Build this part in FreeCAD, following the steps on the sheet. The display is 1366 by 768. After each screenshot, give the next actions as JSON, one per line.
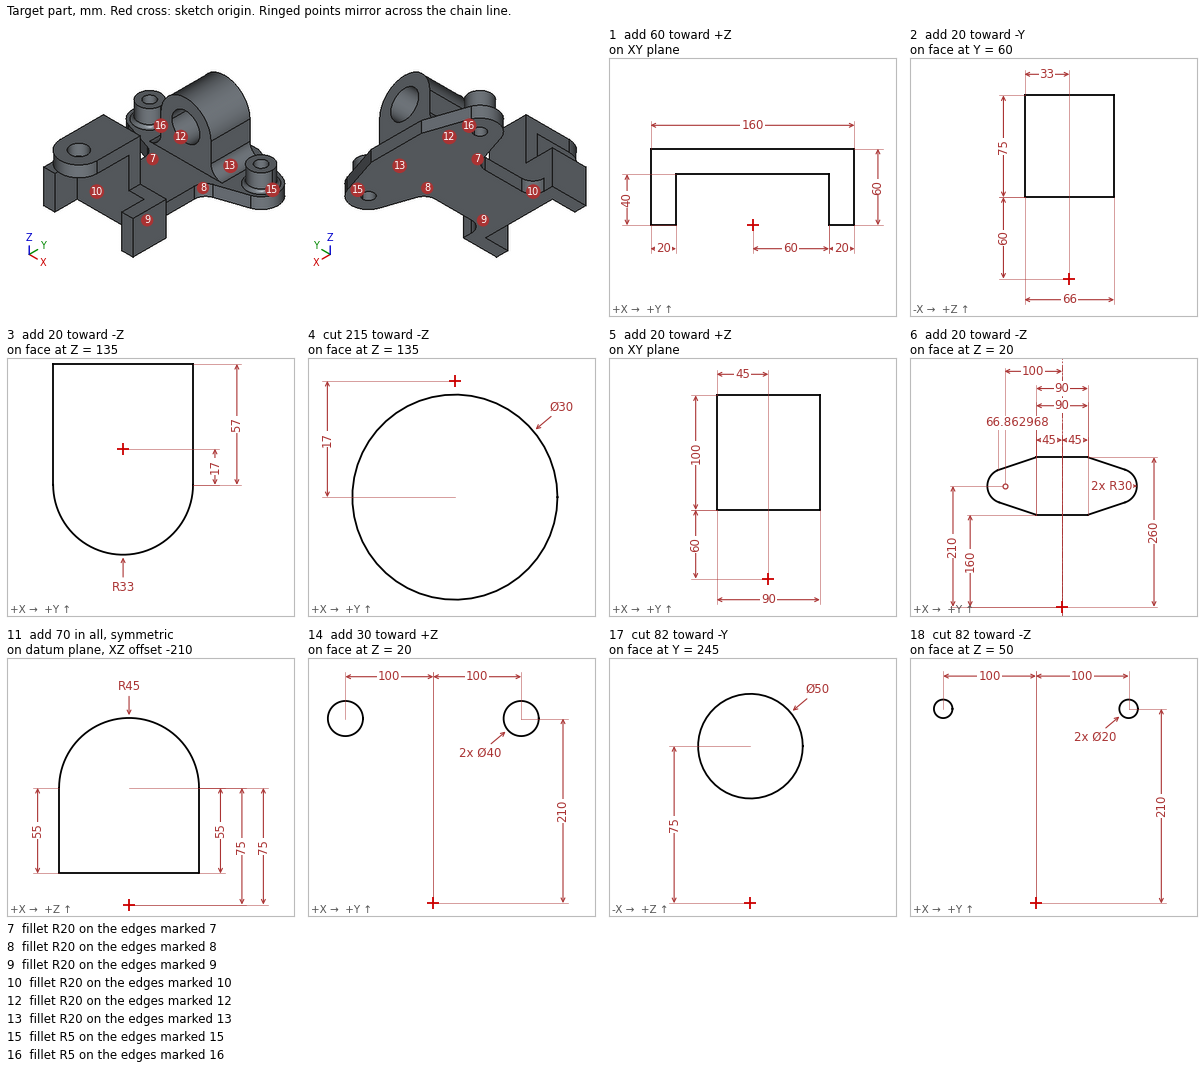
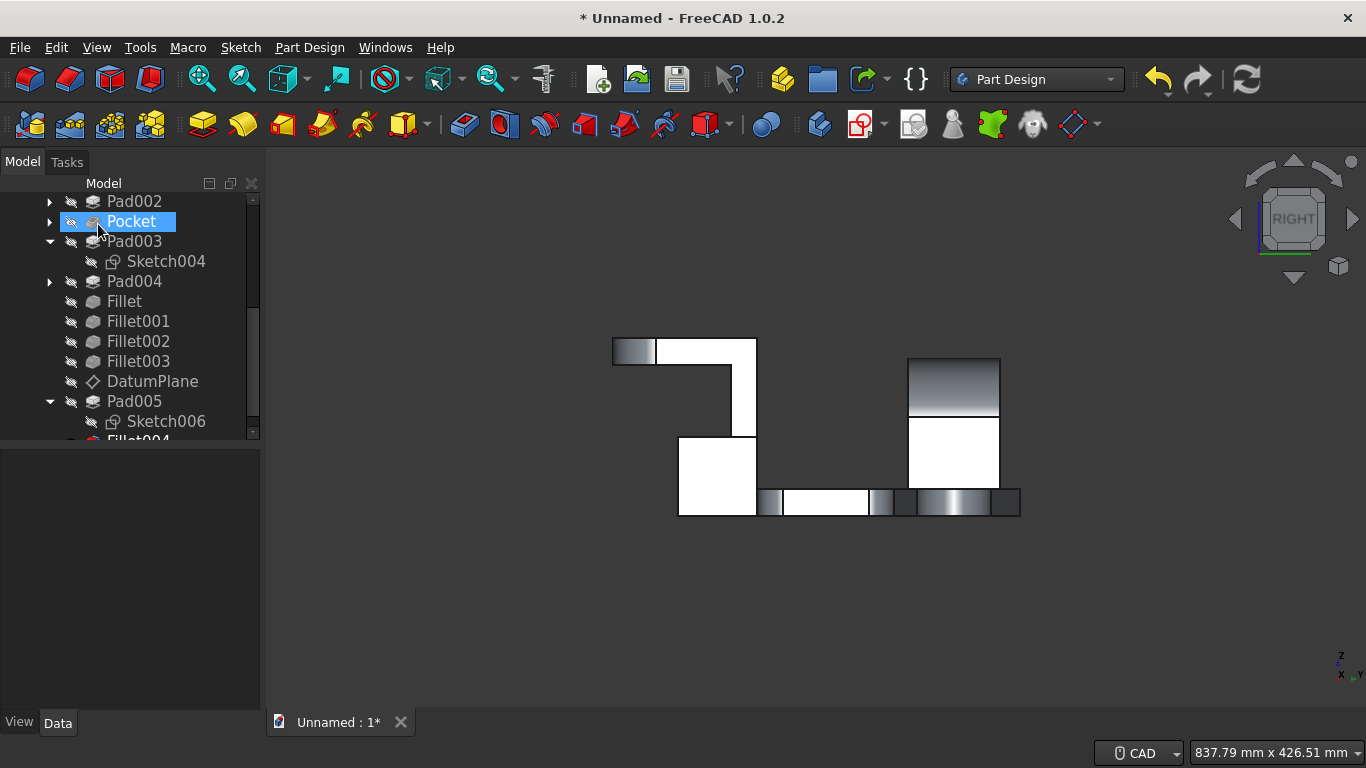
{"action": "key", "text": "v f"}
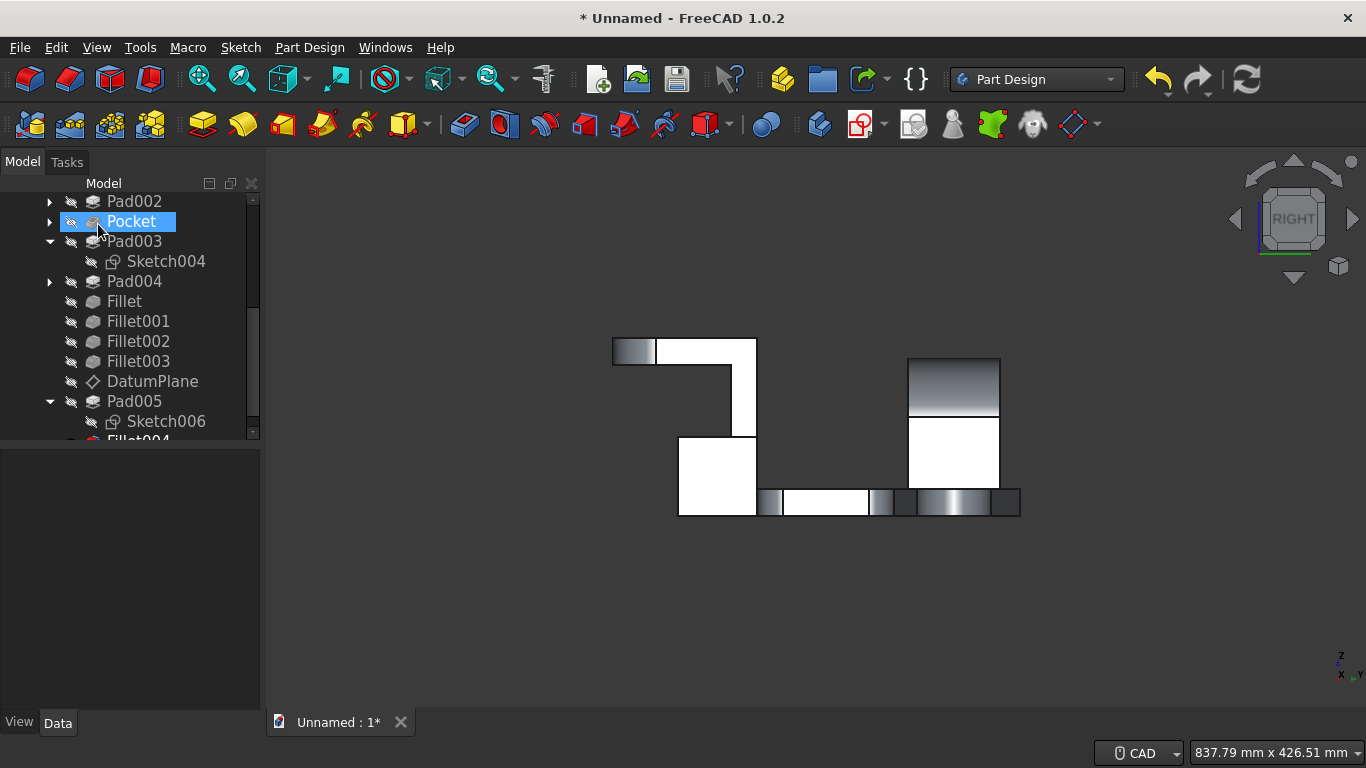
{"action": "key", "text": "5"}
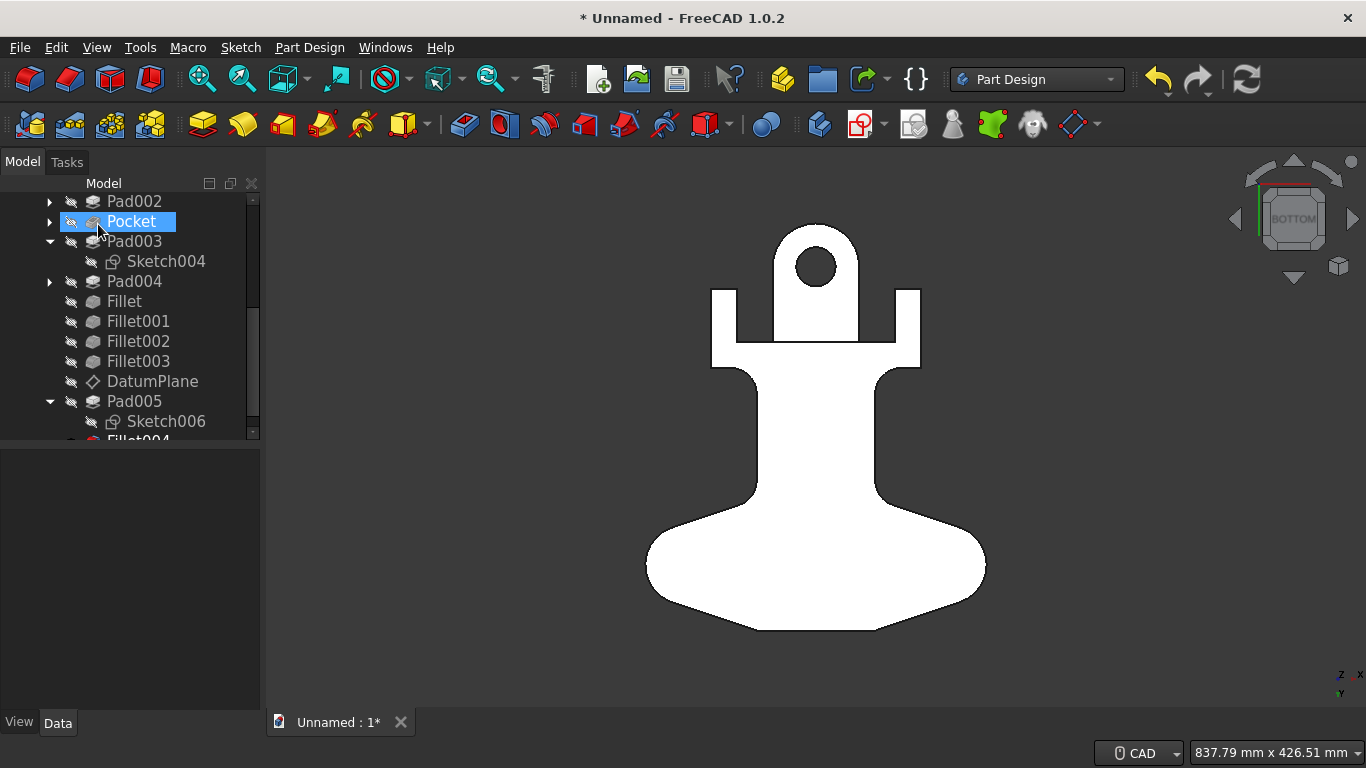
{"action": "key", "text": "4"}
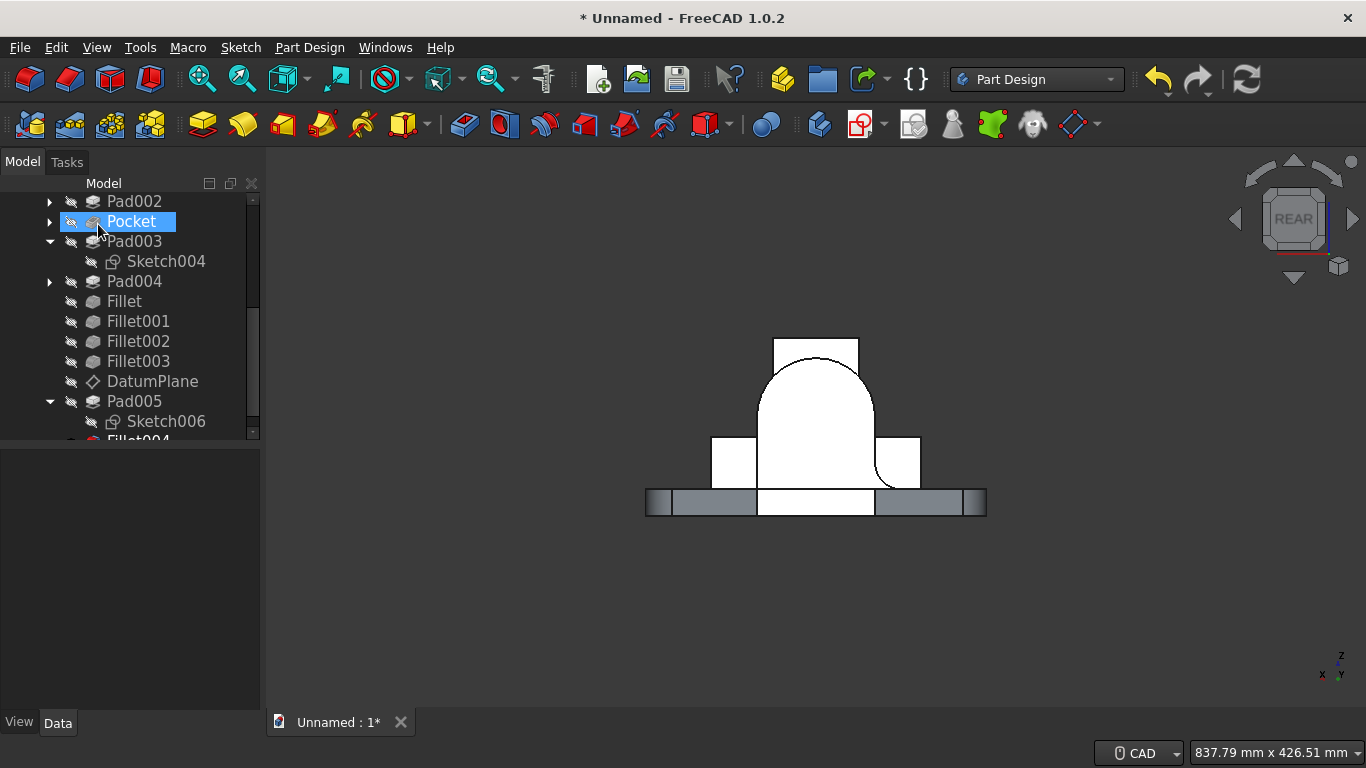
{"action": "key", "text": "v f"}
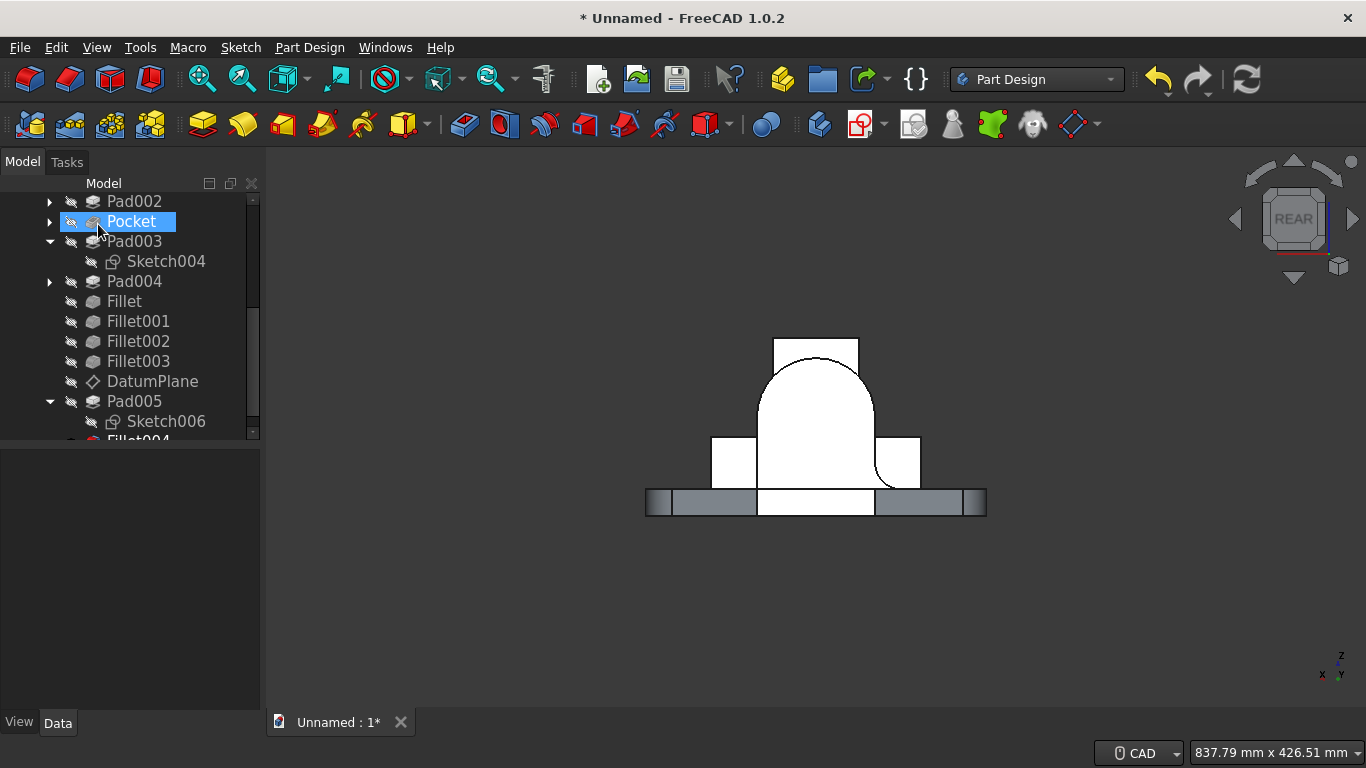
{"action": "key", "text": "6"}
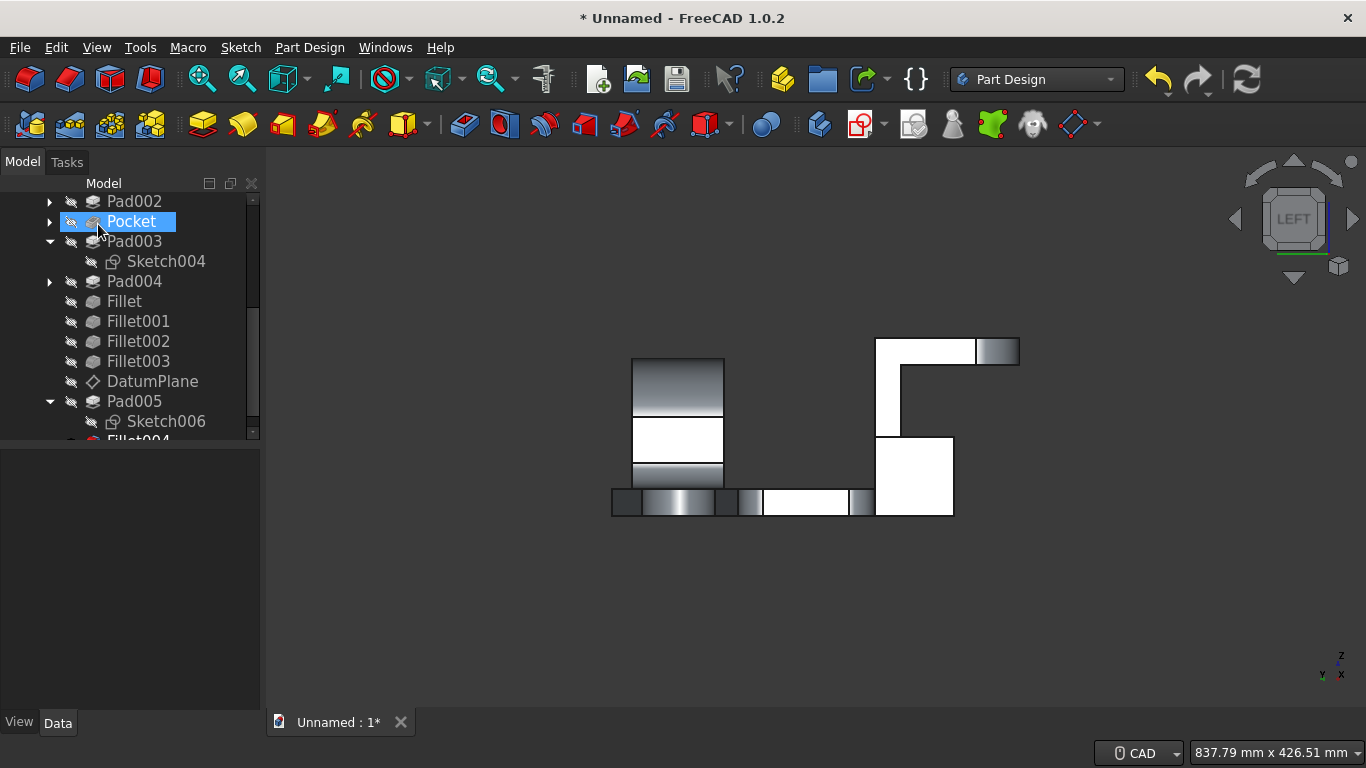
{"action": "left_click", "coordinate": [204, 80]}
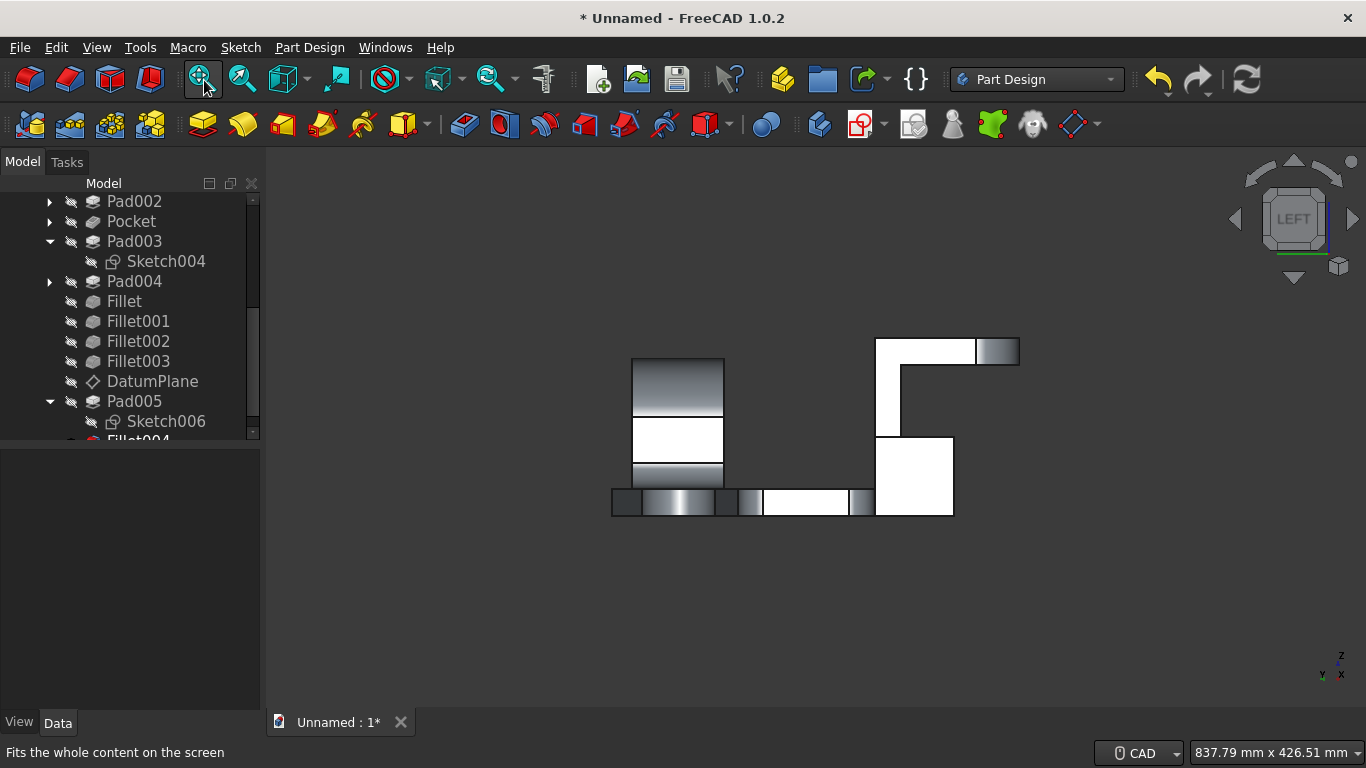
{"action": "key", "text": "v 3"}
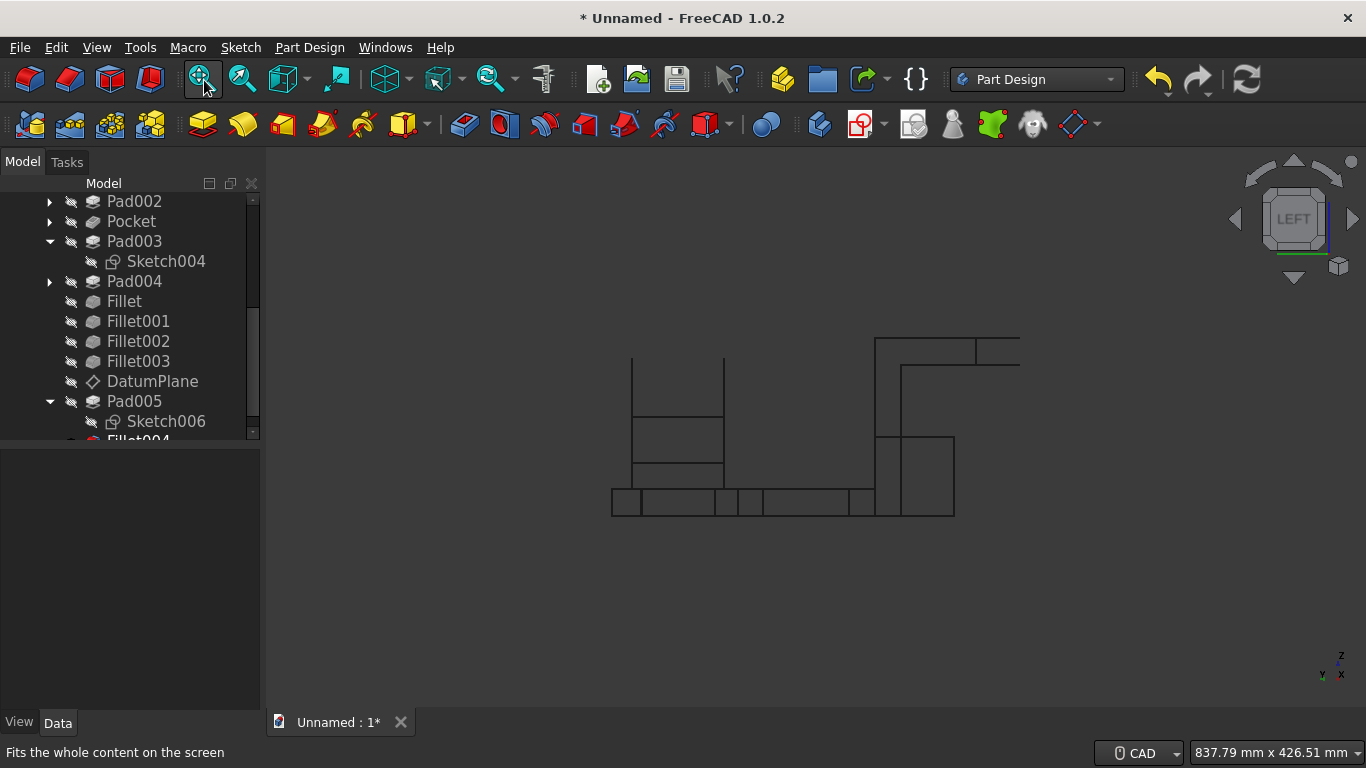
{"action": "key", "text": "0"}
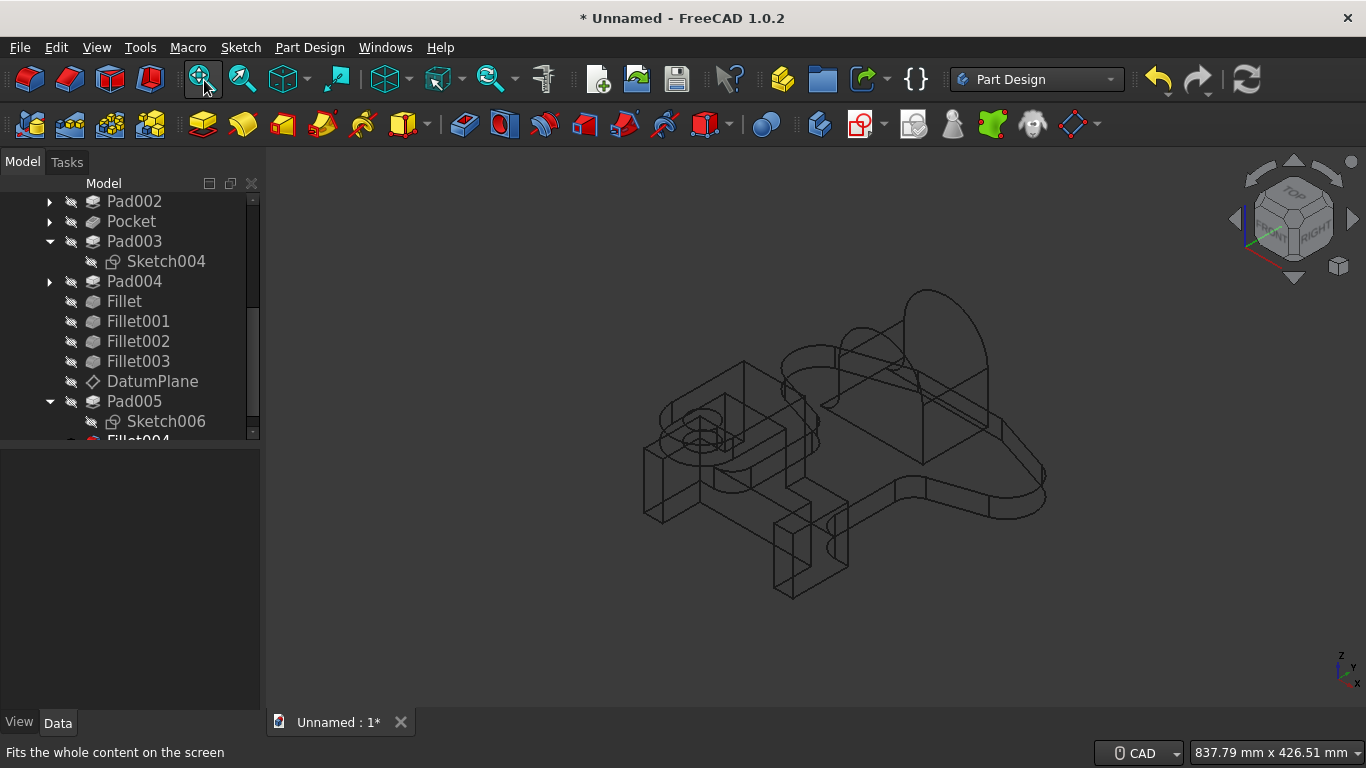
{"action": "left_click", "coordinate": [955, 445]}